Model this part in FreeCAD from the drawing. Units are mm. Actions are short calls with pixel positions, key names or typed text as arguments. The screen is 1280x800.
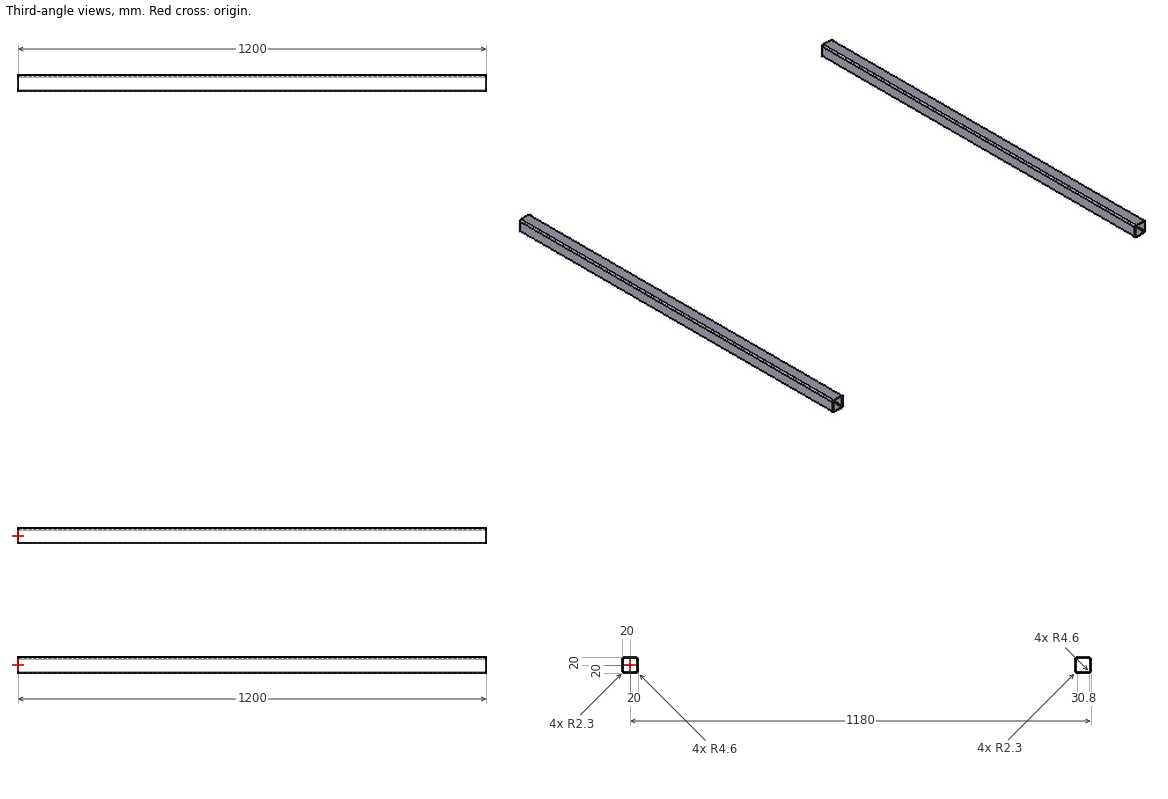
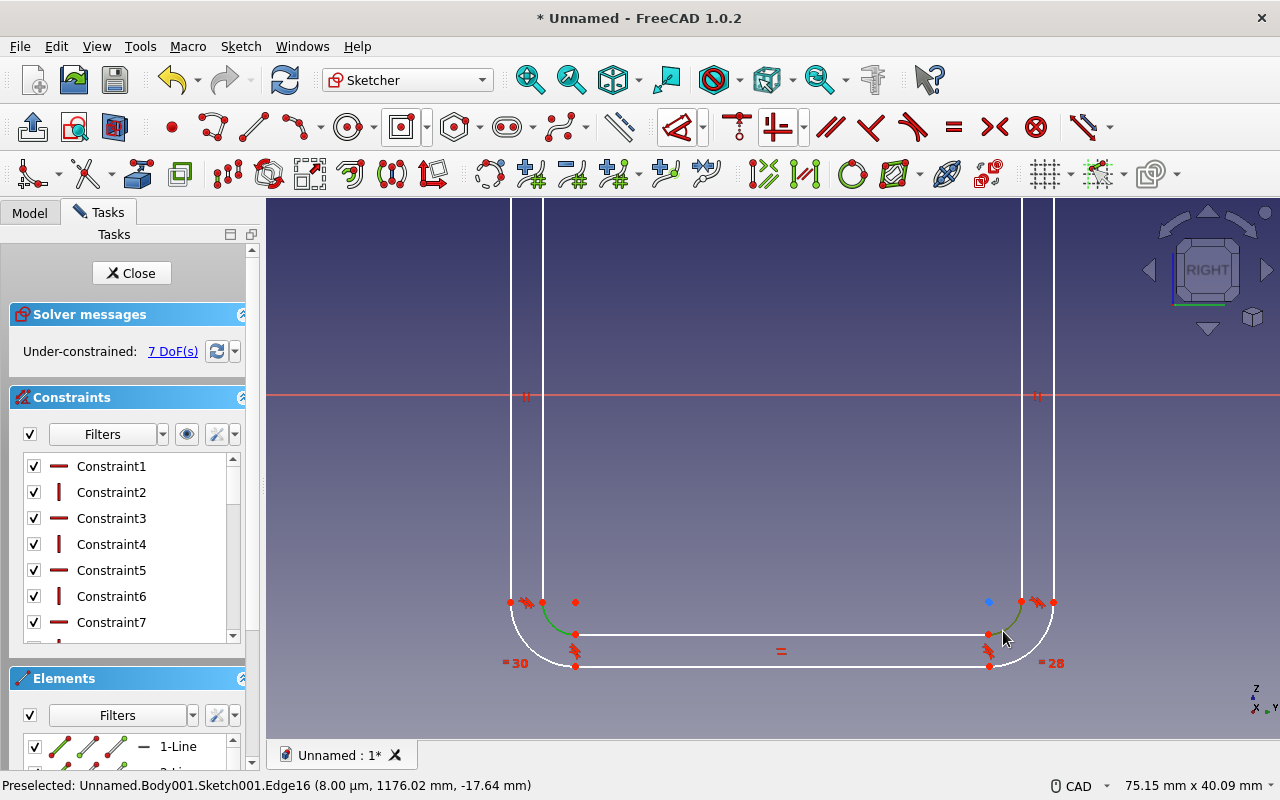
key(e)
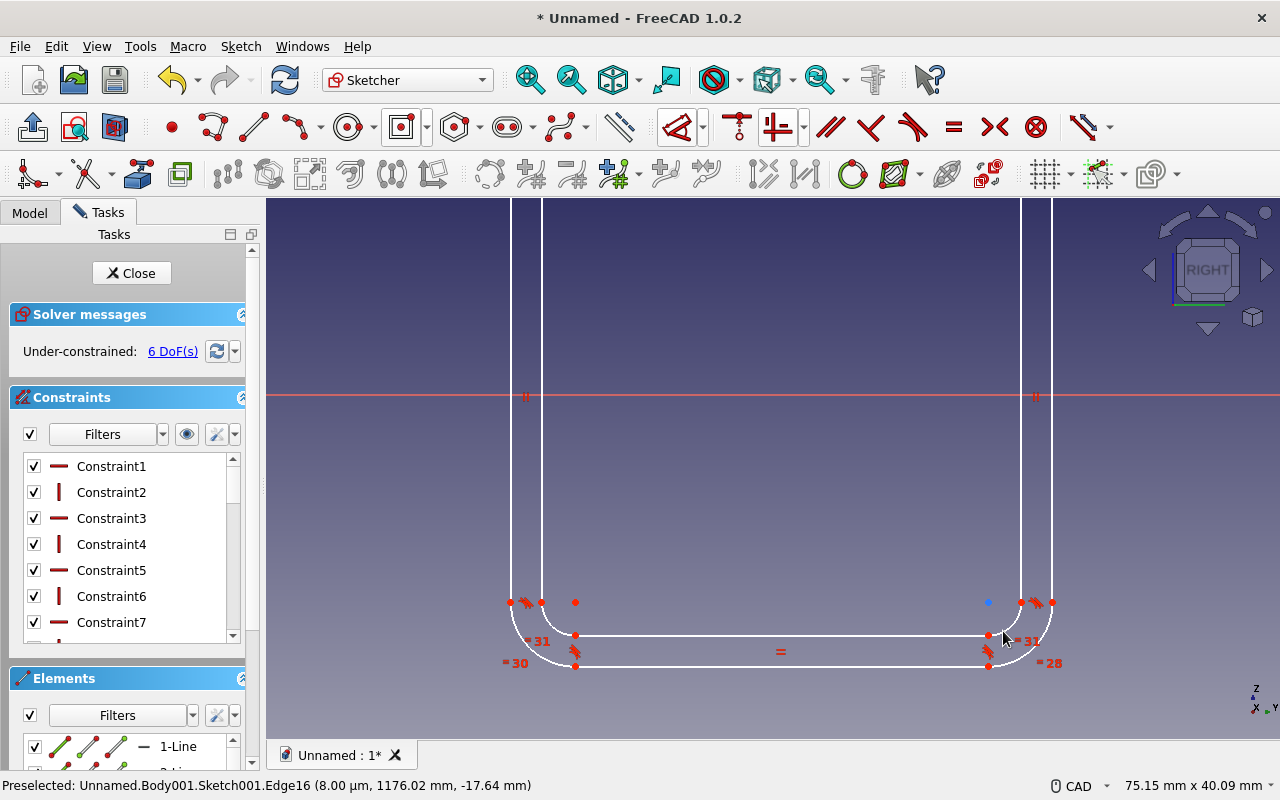
click(1017, 660)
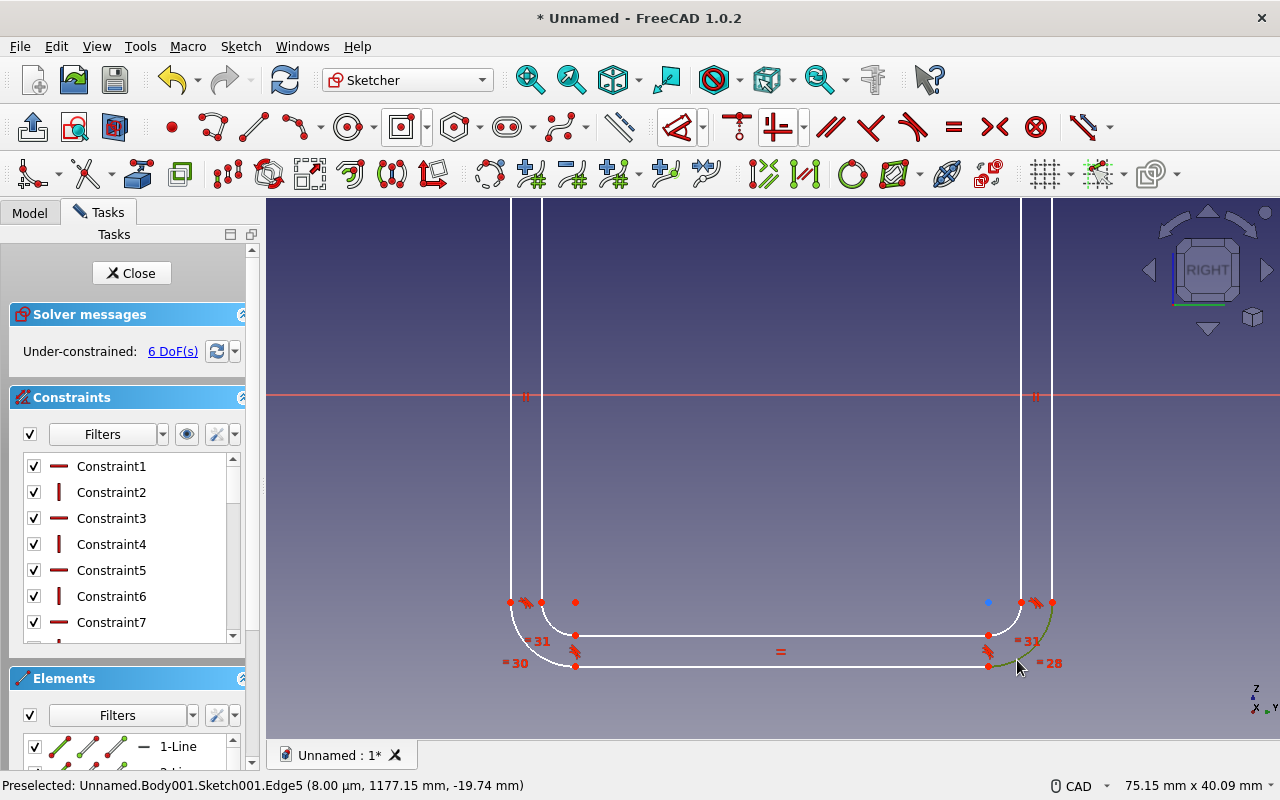
key(k)
key(r)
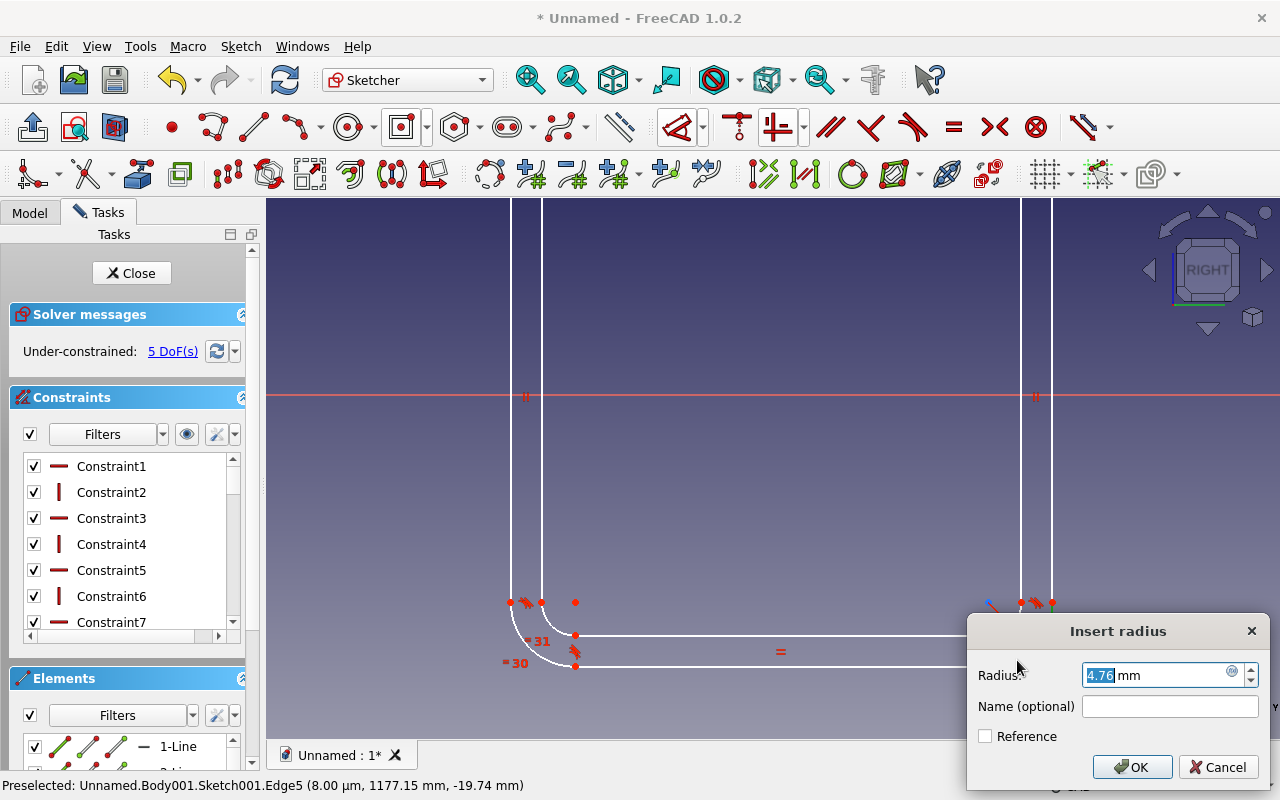
text(4.6)
key(Return)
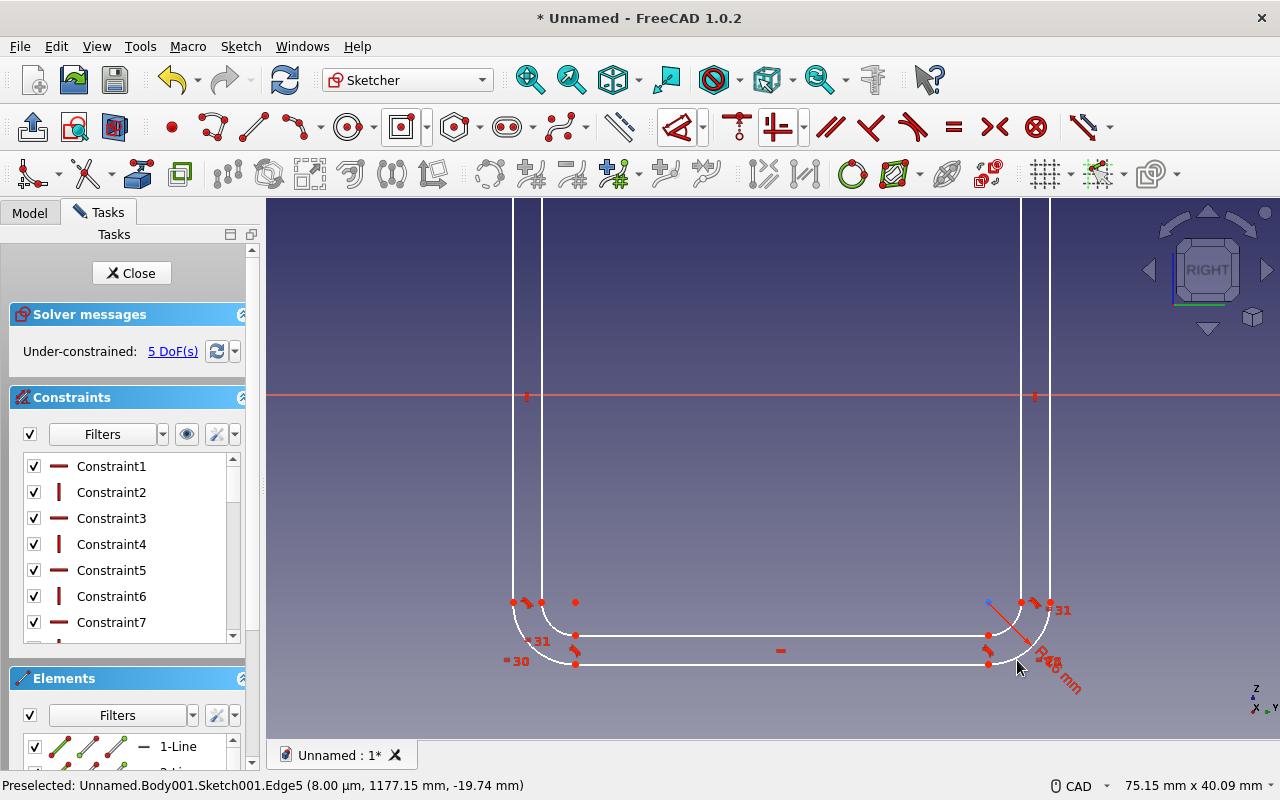
scroll(546, 618, up, 2)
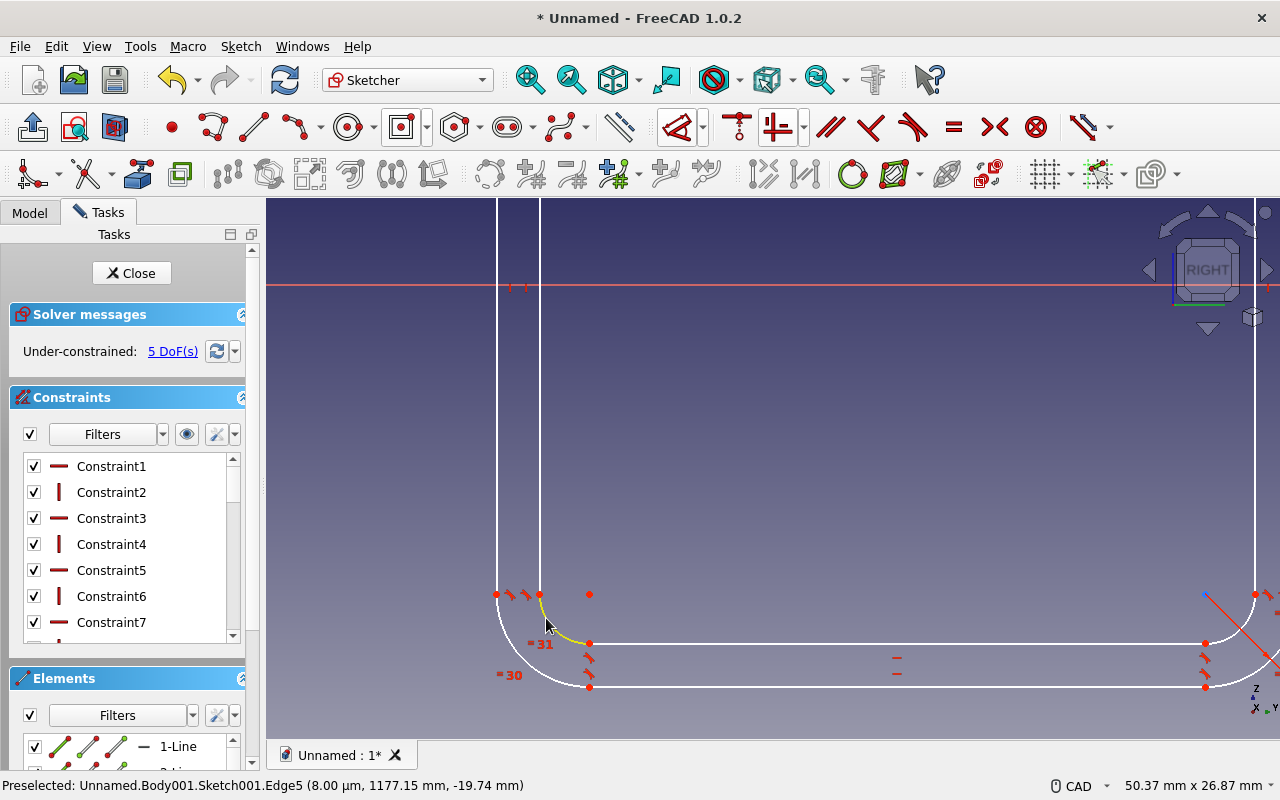
click(545, 617)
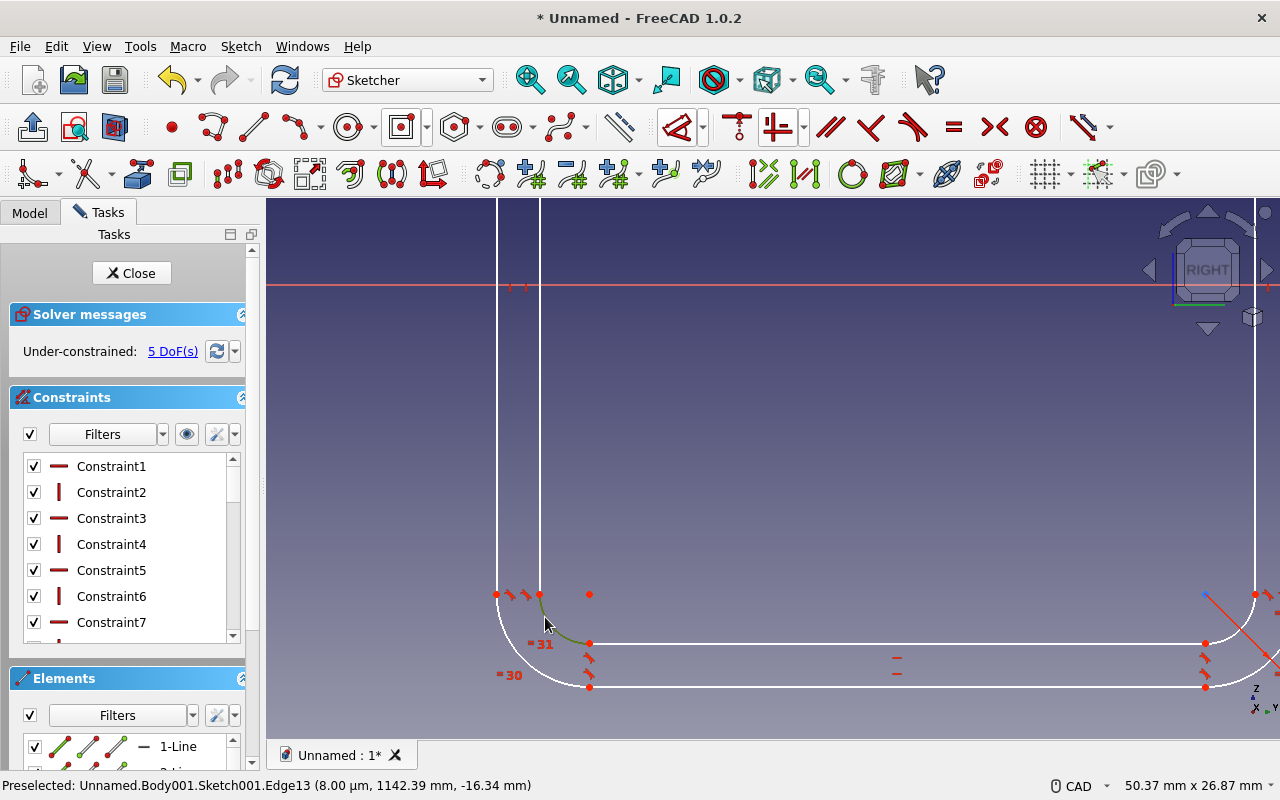
key(k)
key(r)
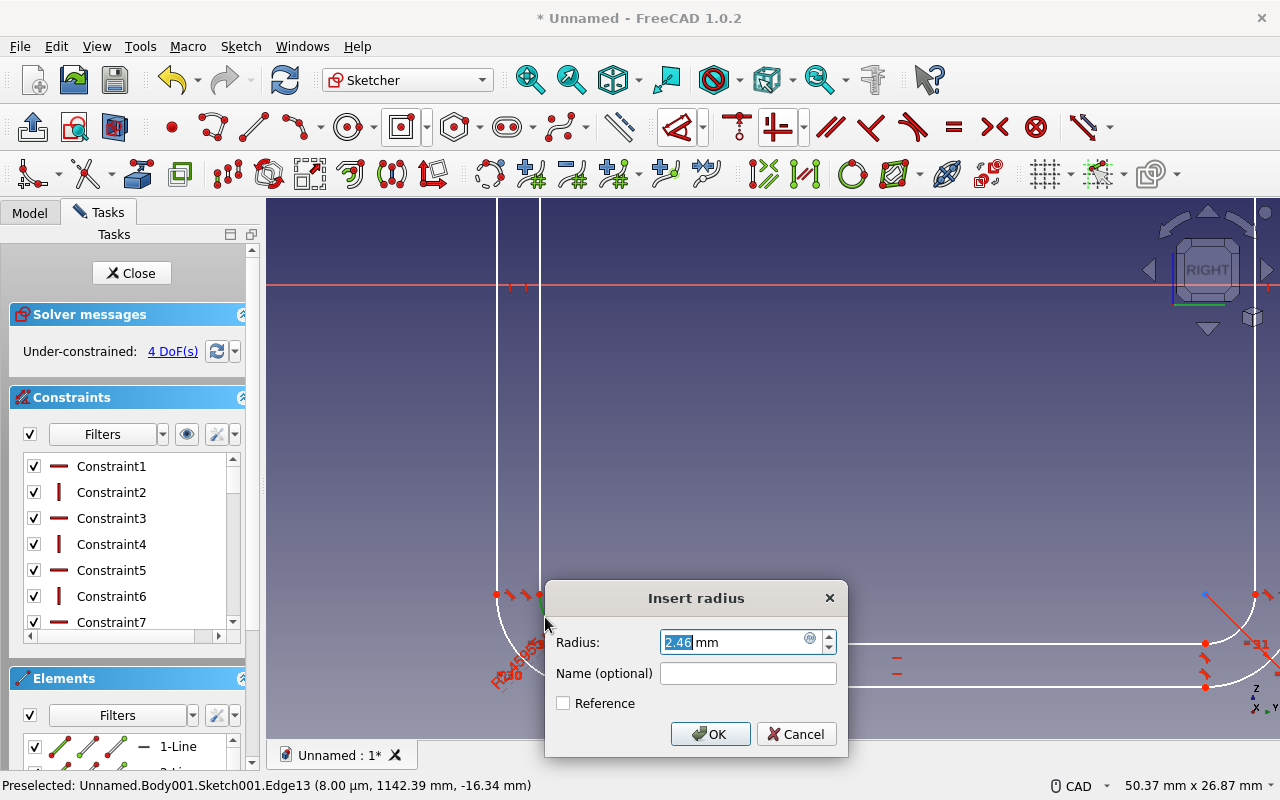
text(2.3)
key(Return)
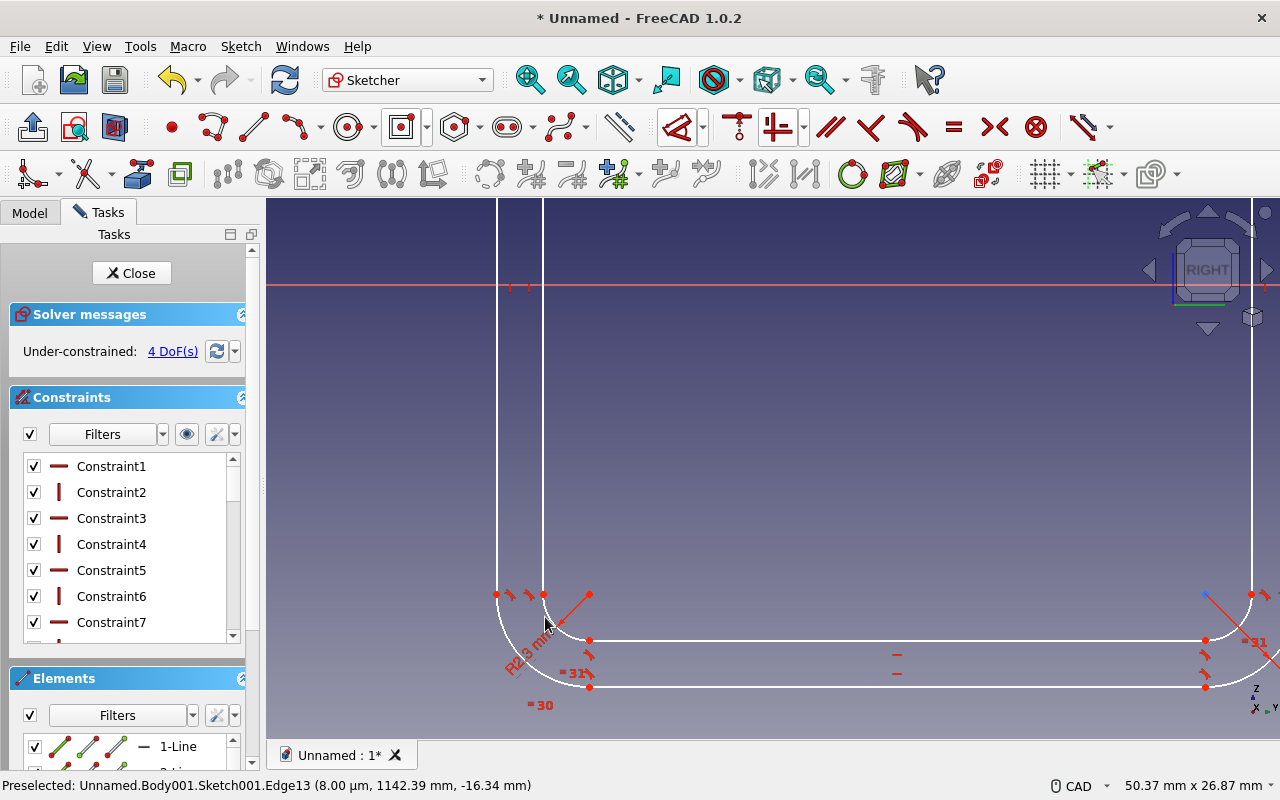
click(589, 687)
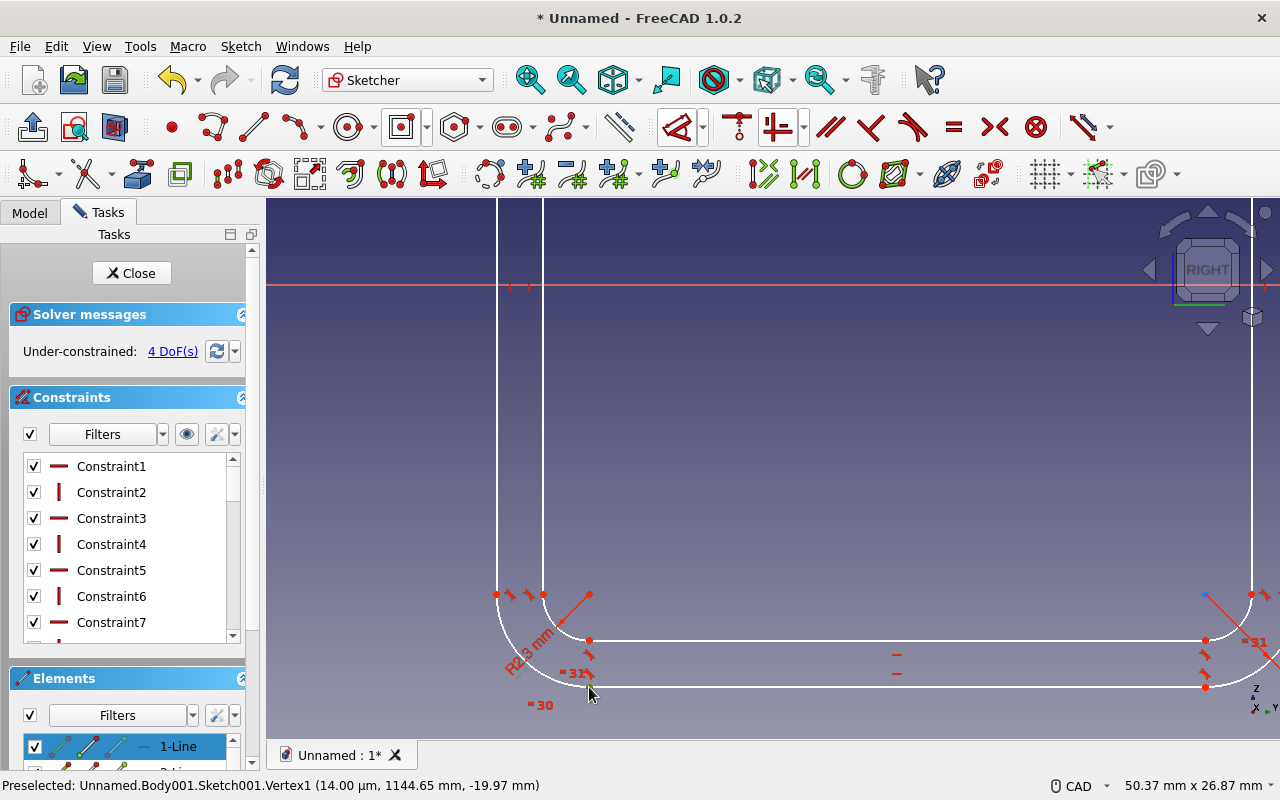
key(i)